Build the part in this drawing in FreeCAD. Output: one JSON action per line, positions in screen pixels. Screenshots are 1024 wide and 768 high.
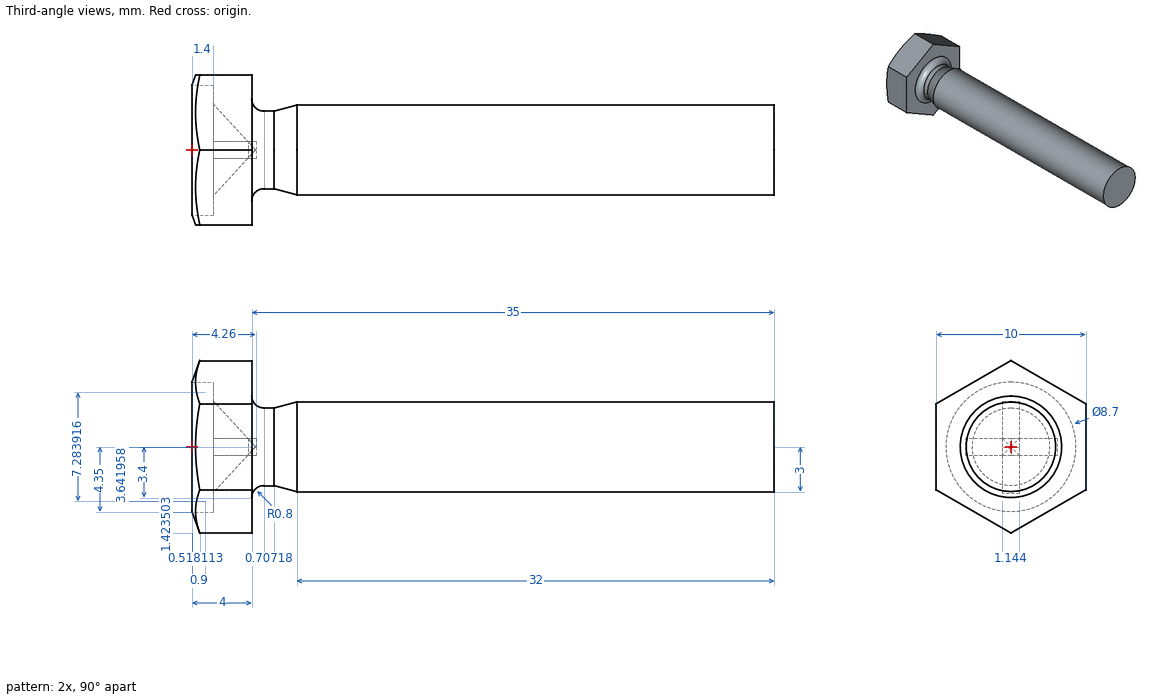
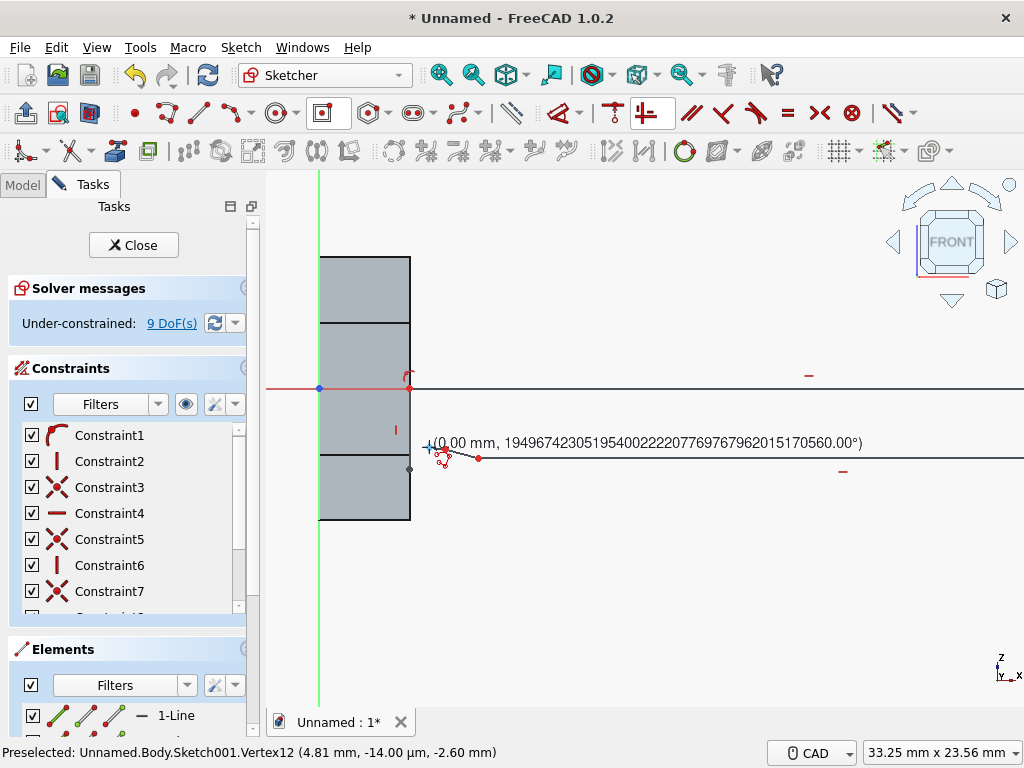
{"action": "left_click", "coordinate": [232, 114]}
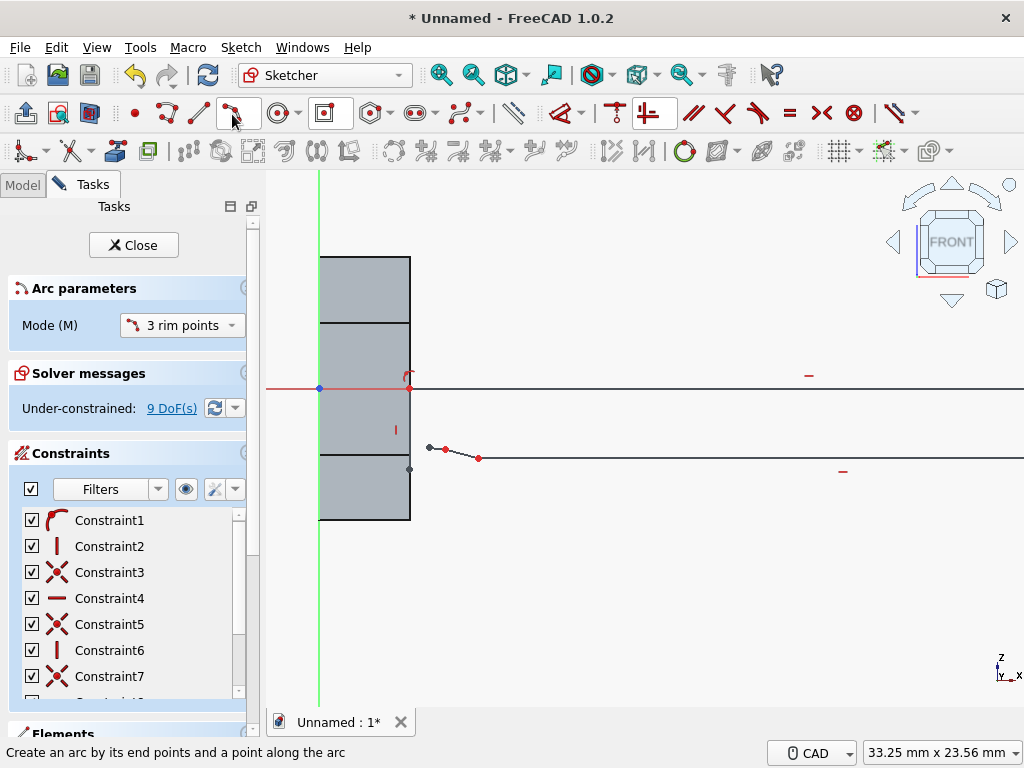
{"action": "scroll", "coordinate": [429, 448], "scroll_direction": "up", "scroll_amount": 4}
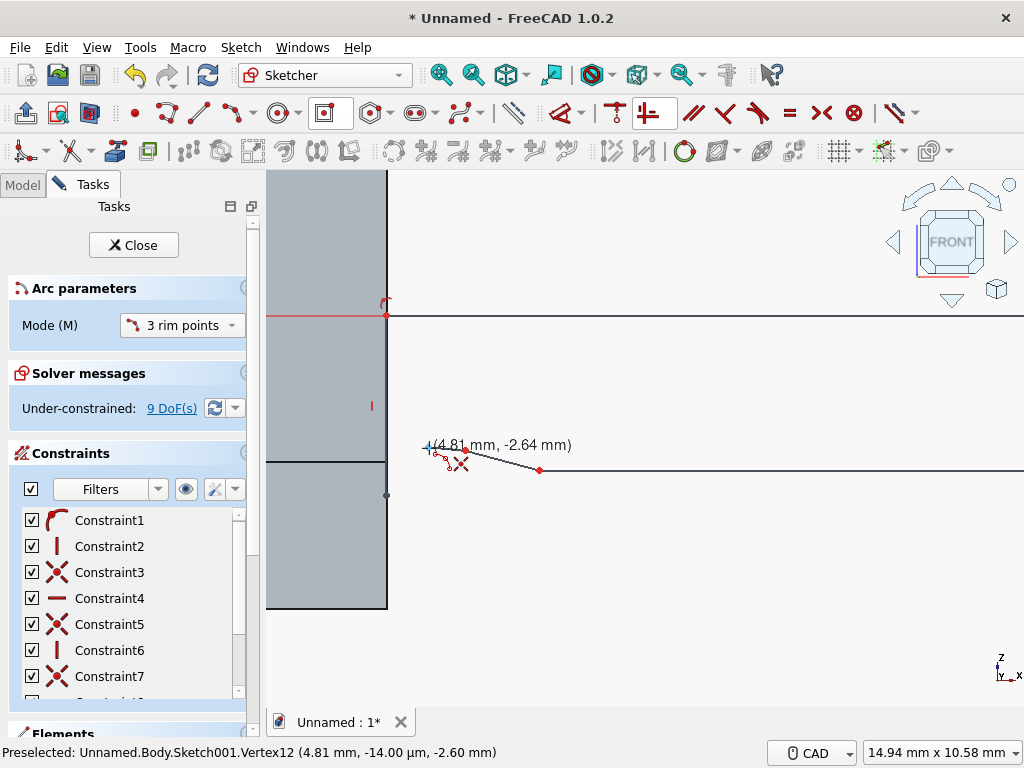
{"action": "left_click", "coordinate": [429, 447]}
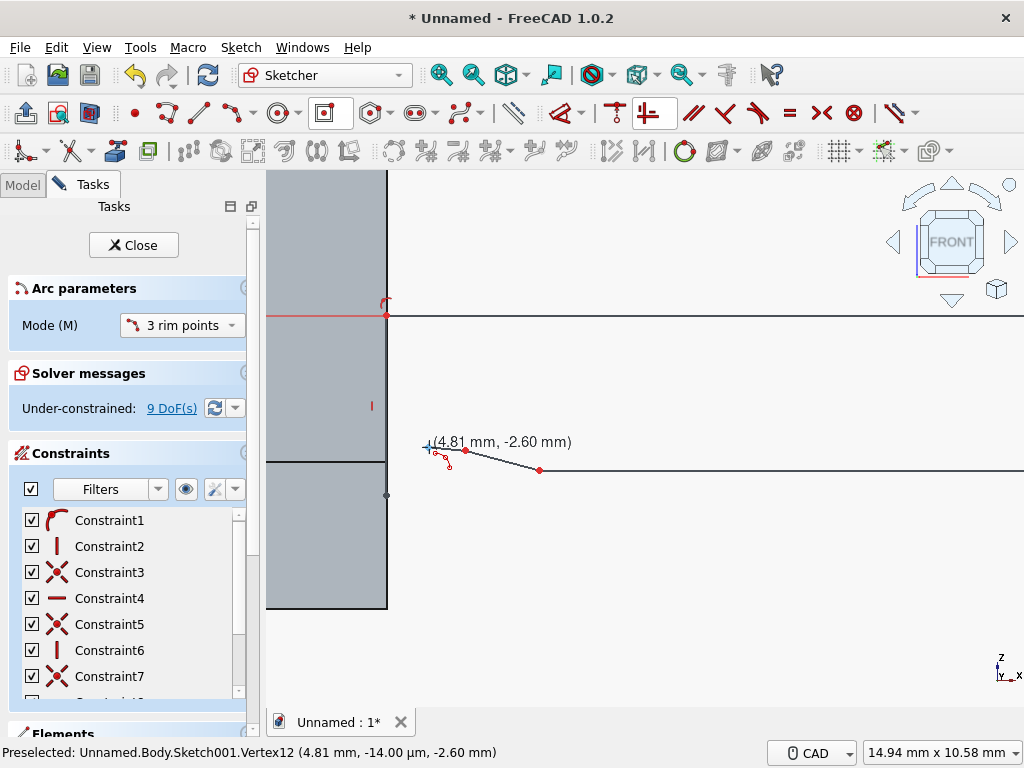
{"action": "scroll", "coordinate": [425, 448], "scroll_direction": "down", "scroll_amount": 8}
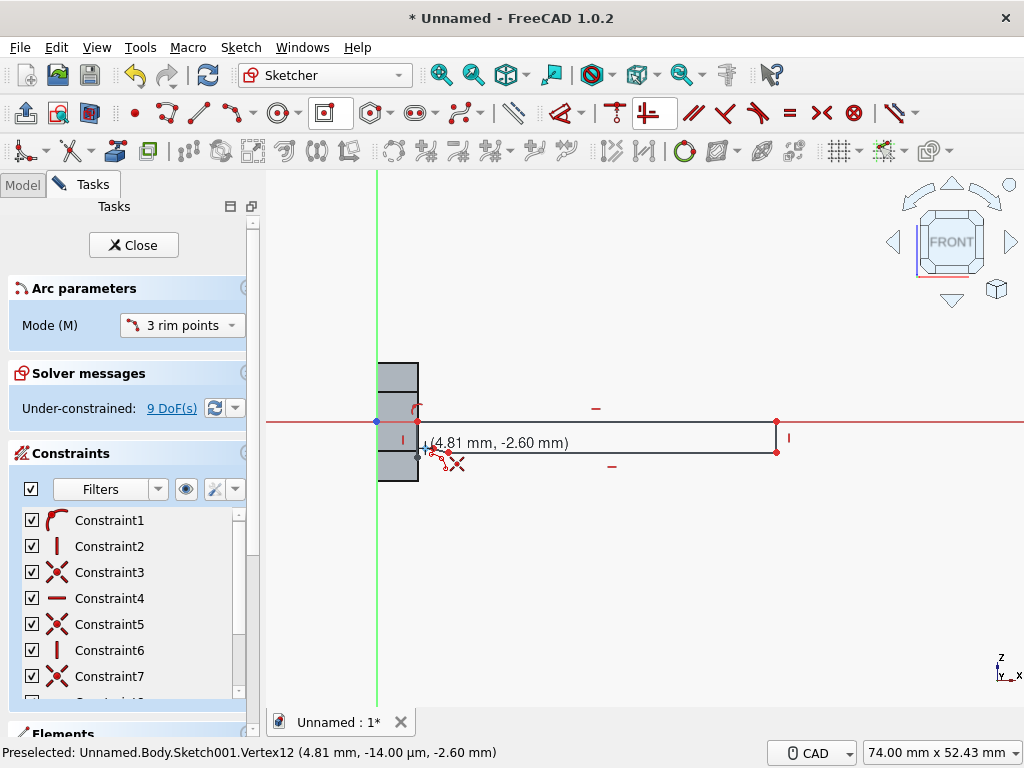
{"action": "scroll", "coordinate": [418, 457], "scroll_direction": "up", "scroll_amount": 2}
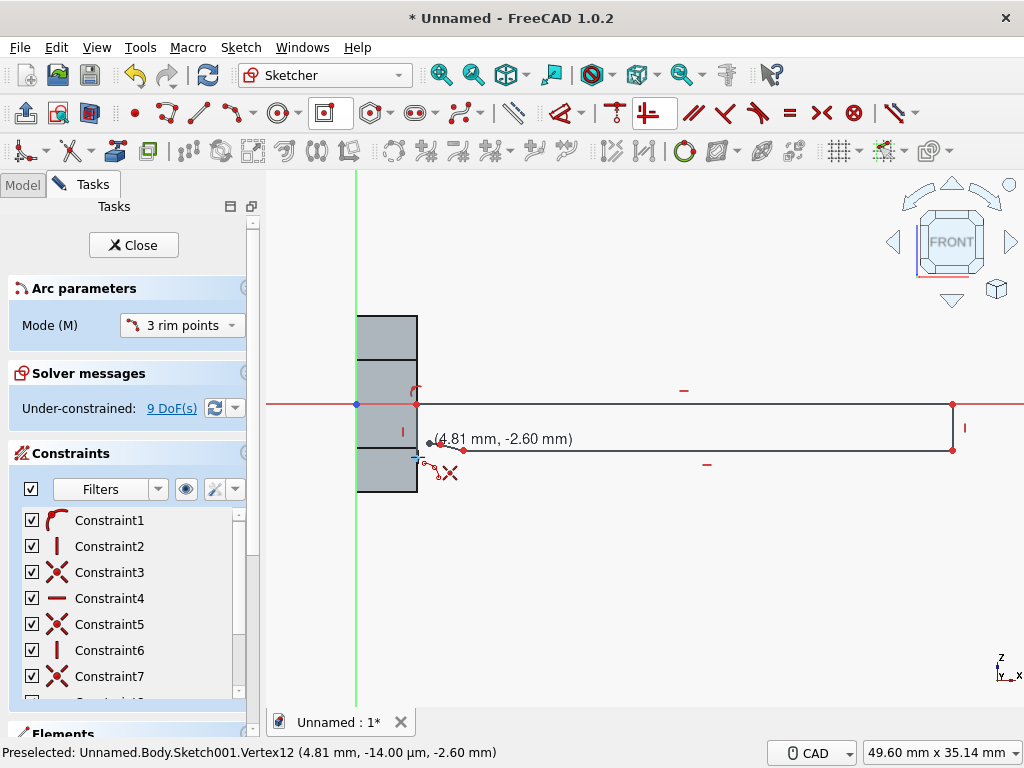
{"action": "left_click", "coordinate": [417, 458]}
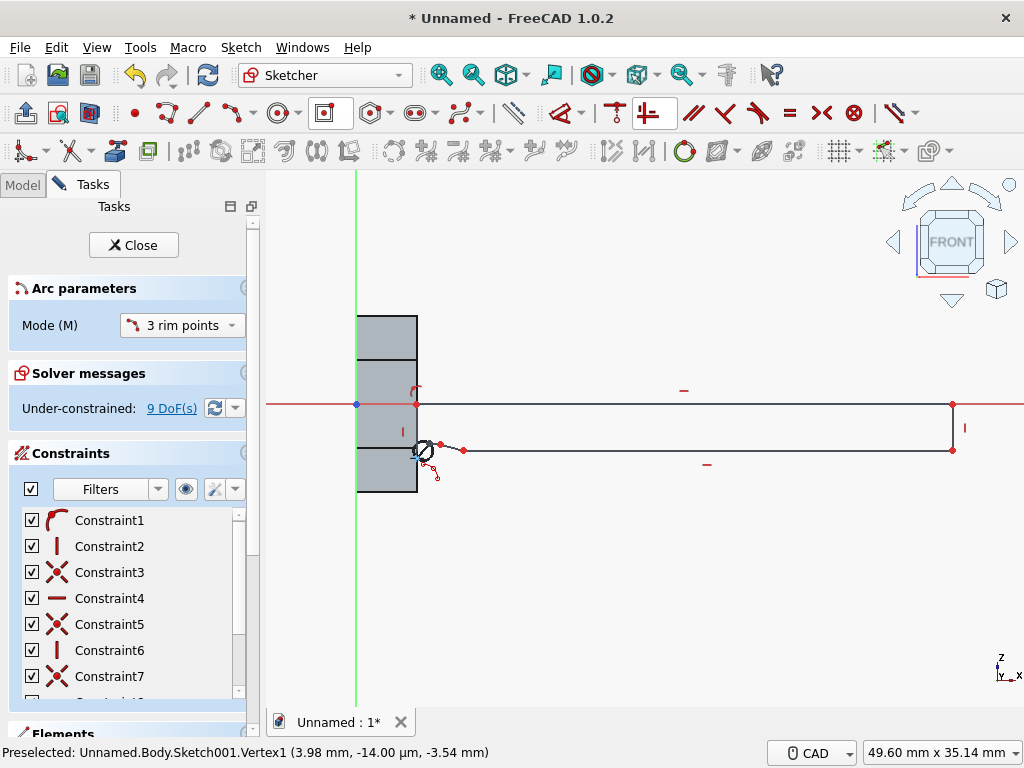
{"action": "scroll", "coordinate": [421, 447], "scroll_direction": "up", "scroll_amount": 8}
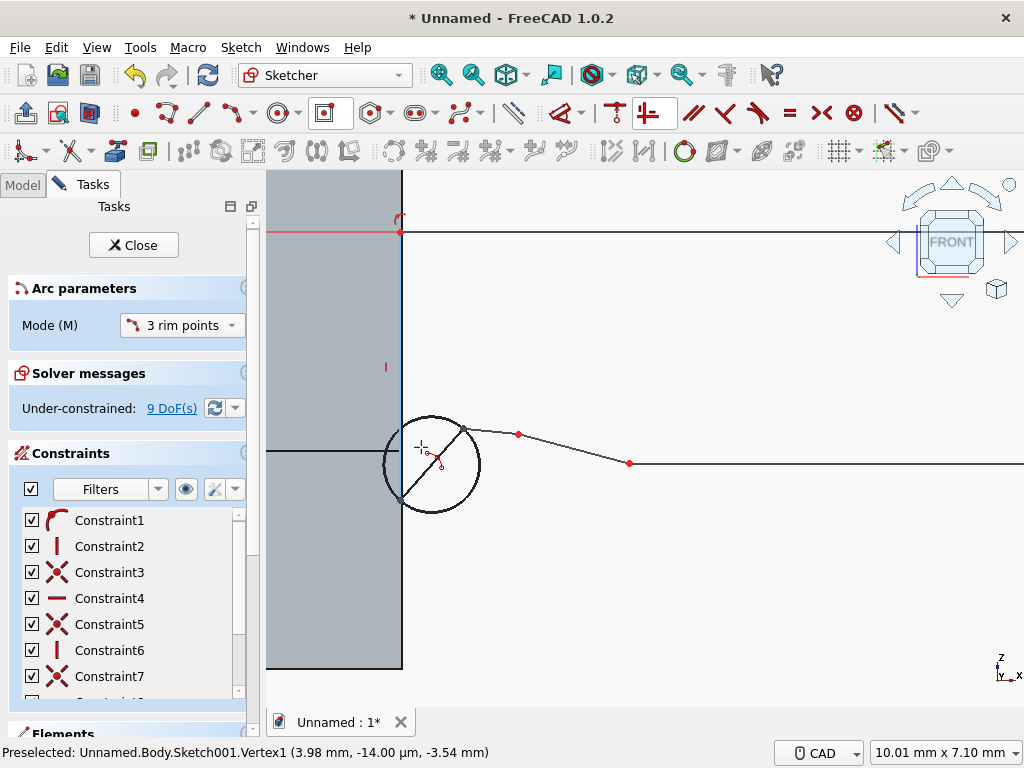
{"action": "left_click", "coordinate": [420, 447]}
{"action": "key", "text": "Escape"}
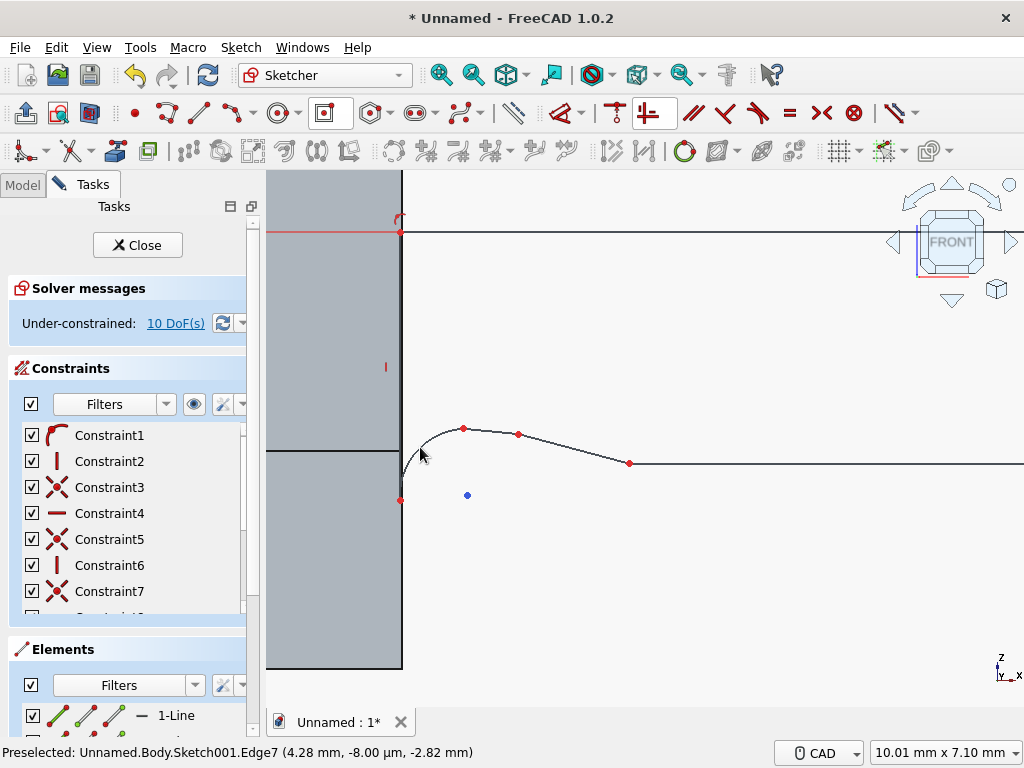
{"action": "left_click", "coordinate": [400, 420]}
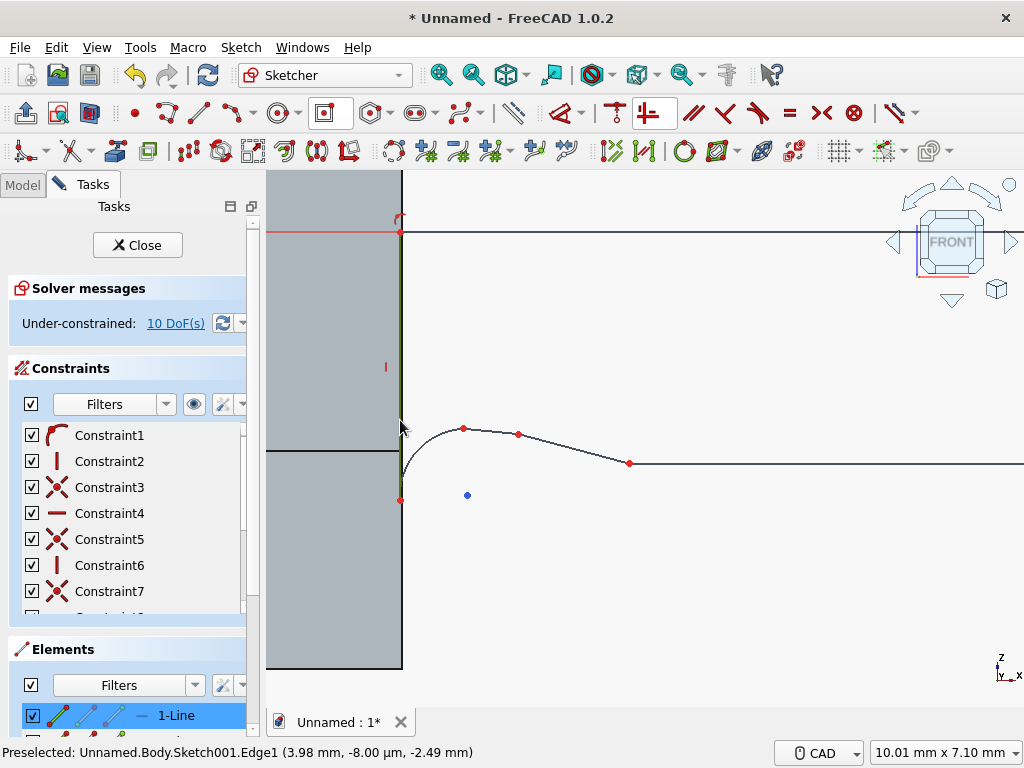
{"action": "left_click", "coordinate": [433, 438]}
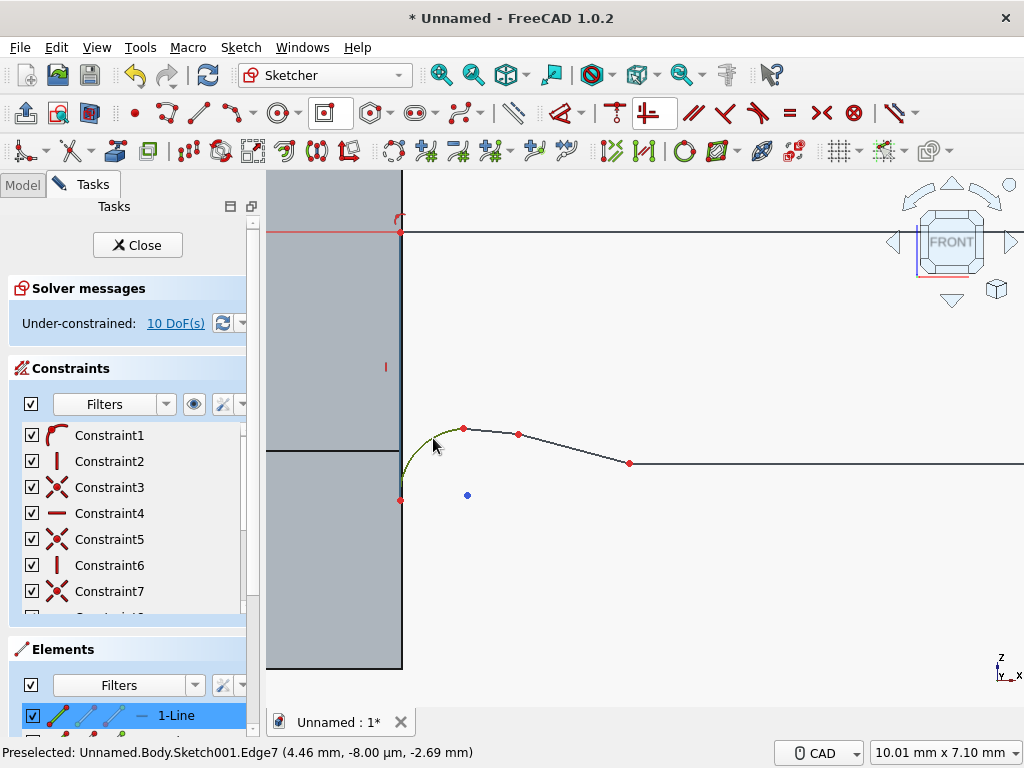
{"action": "left_click", "coordinate": [758, 114]}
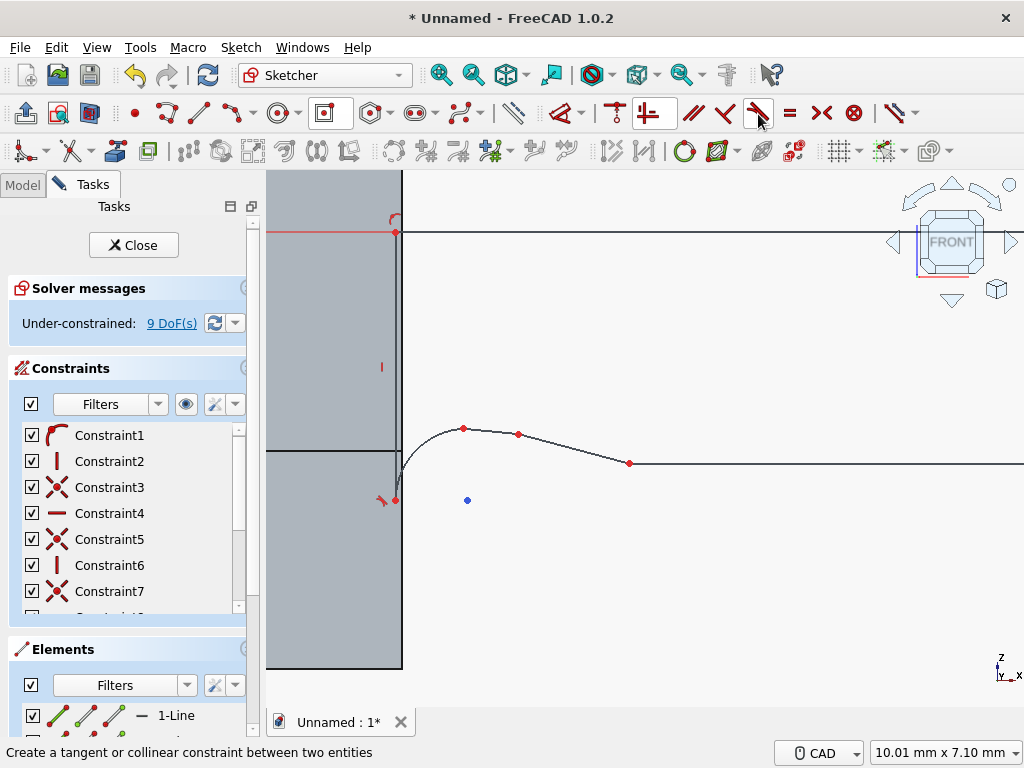
{"action": "left_click", "coordinate": [502, 432]}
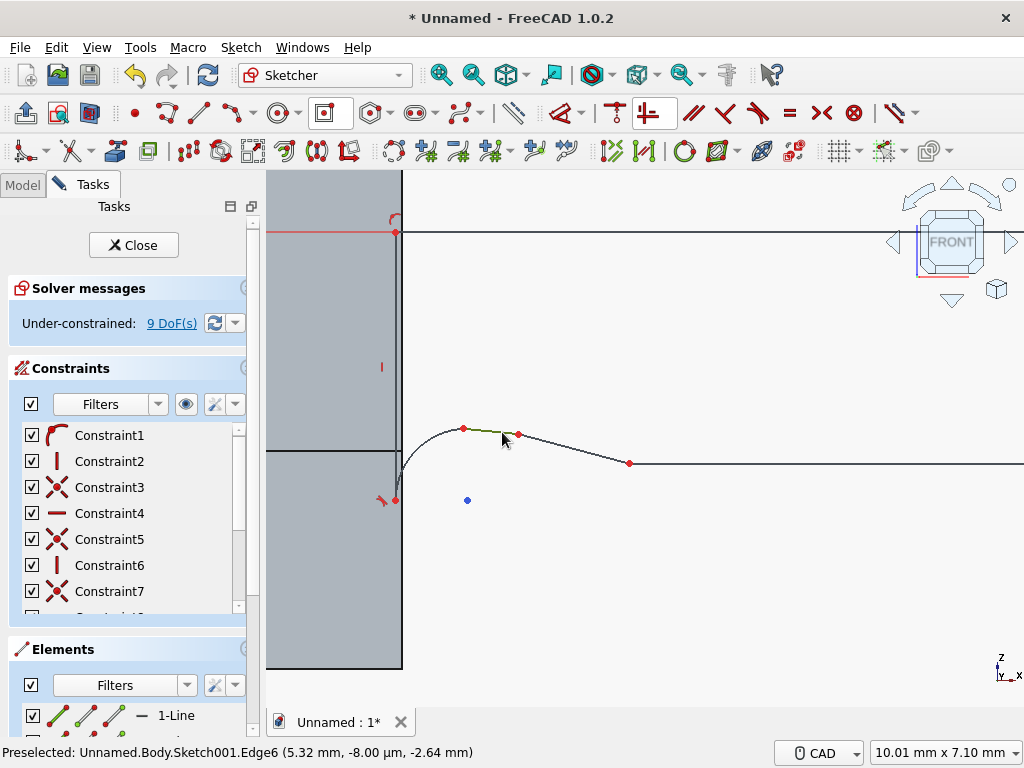
{"action": "left_click", "coordinate": [432, 438]}